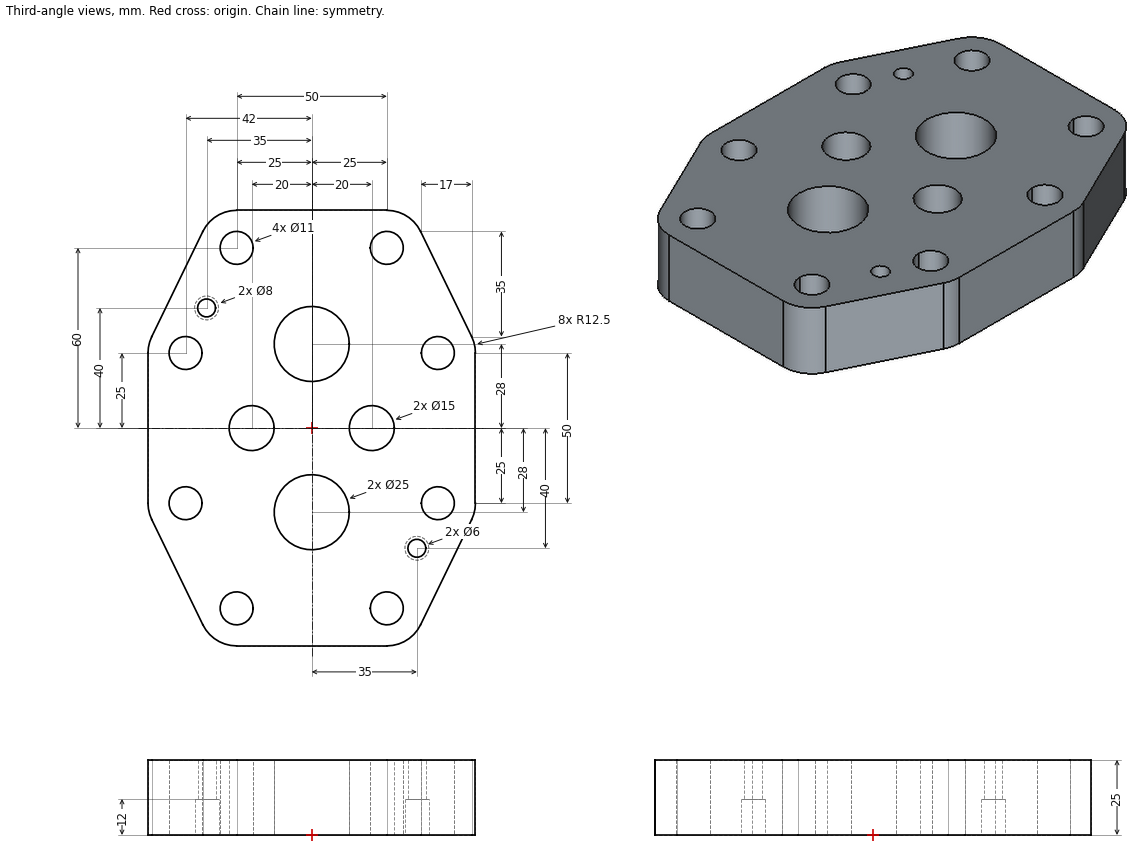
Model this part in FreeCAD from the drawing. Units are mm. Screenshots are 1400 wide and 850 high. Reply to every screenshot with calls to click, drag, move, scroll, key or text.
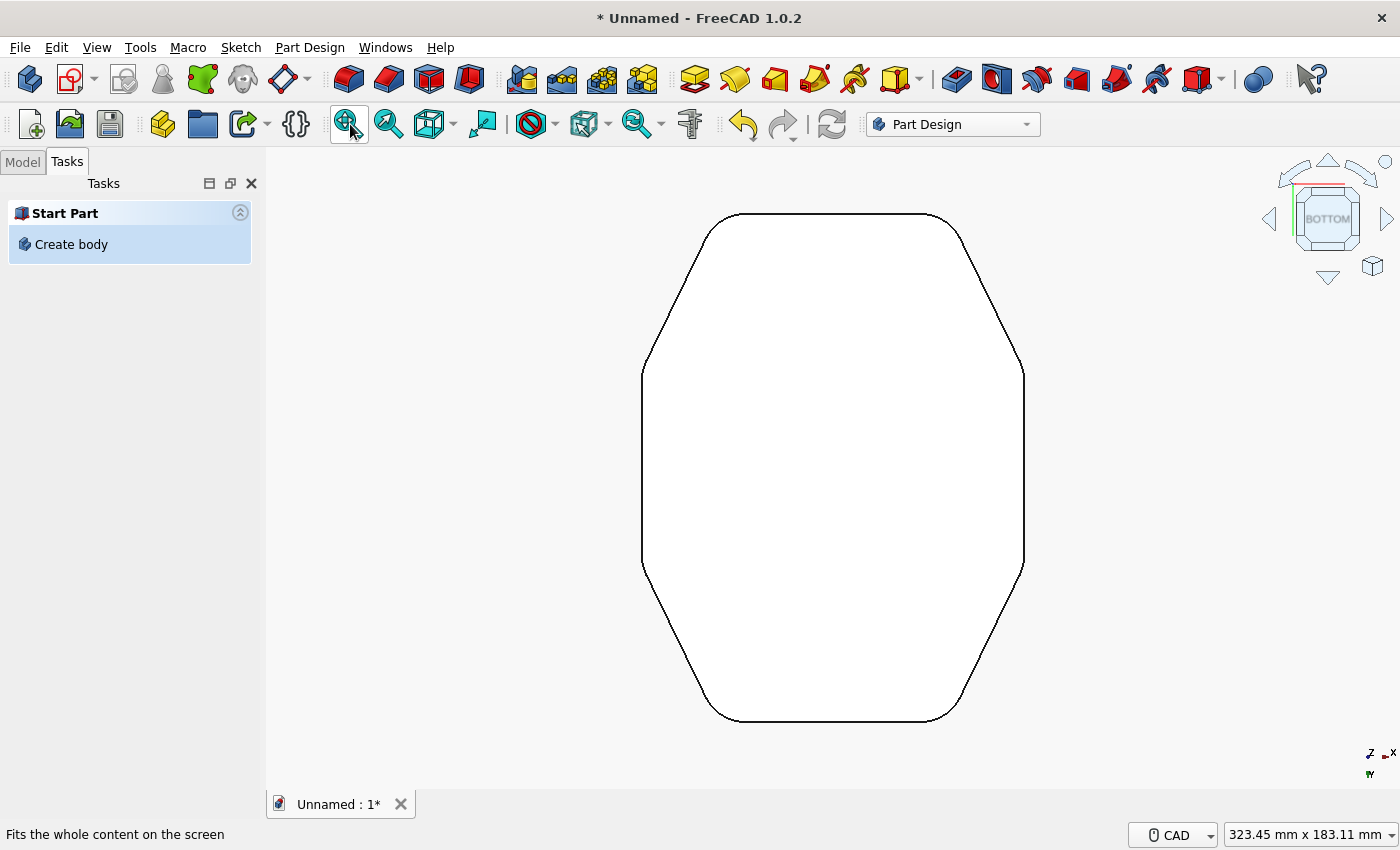
click(833, 467)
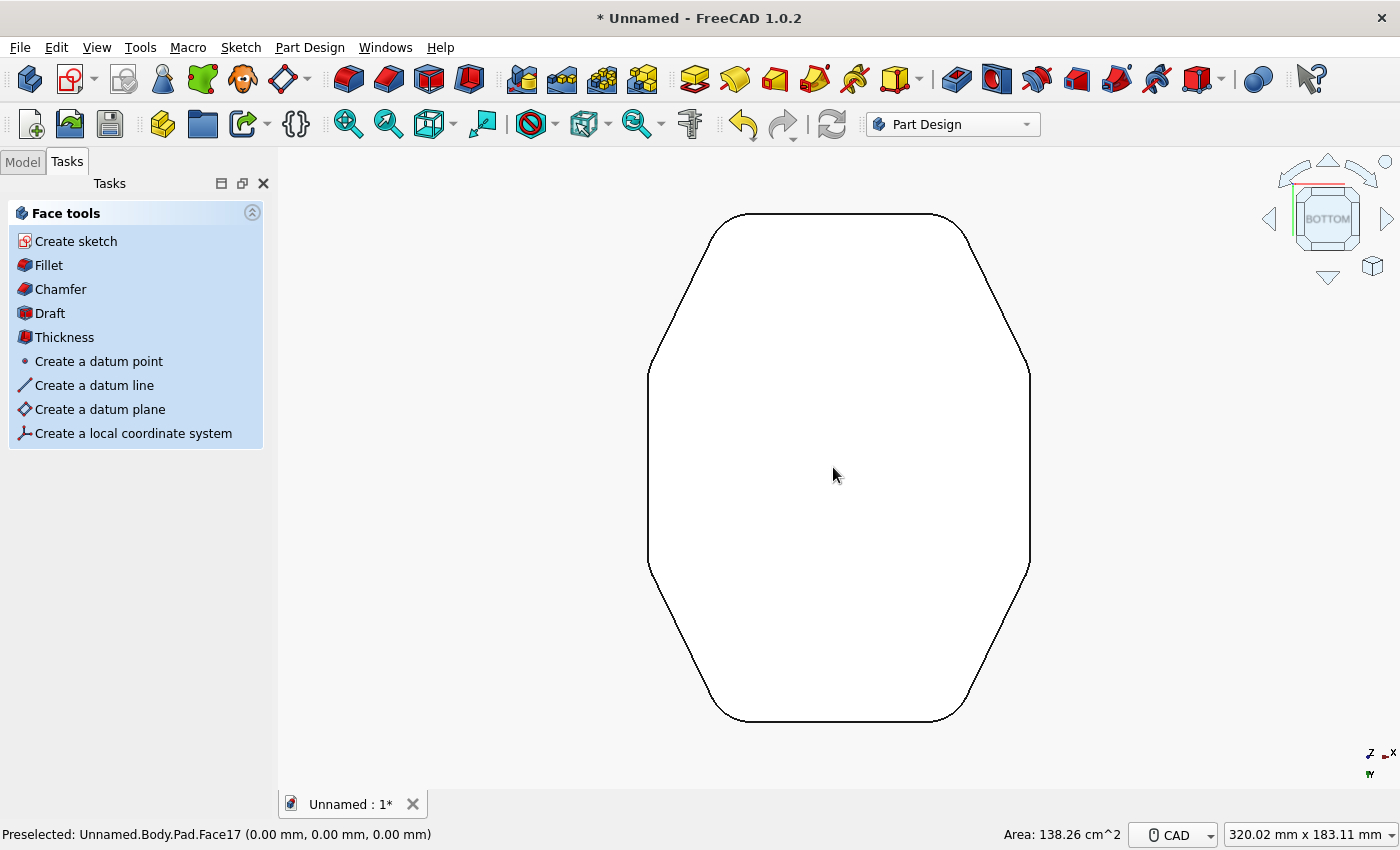
click(70, 80)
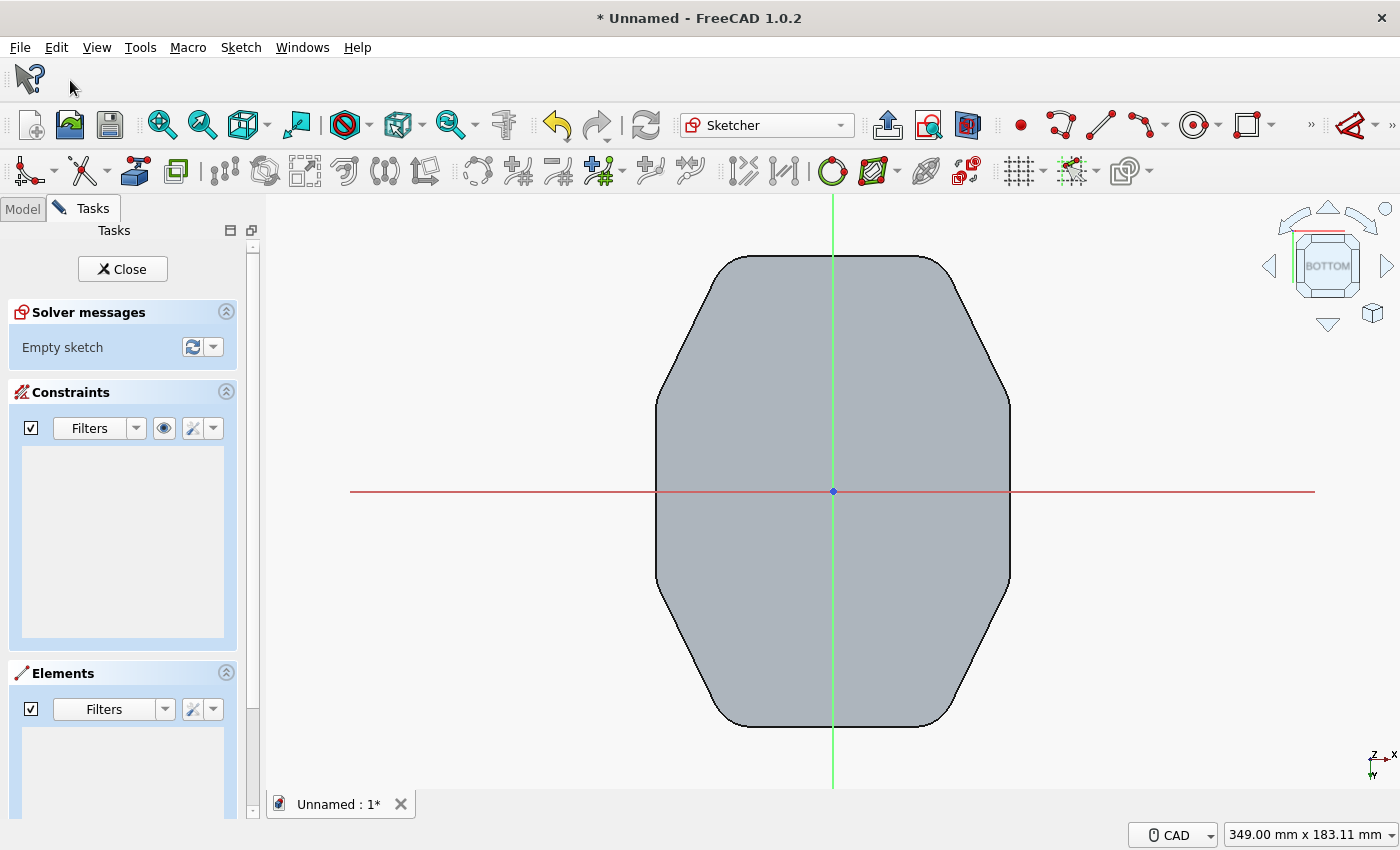
click(1194, 126)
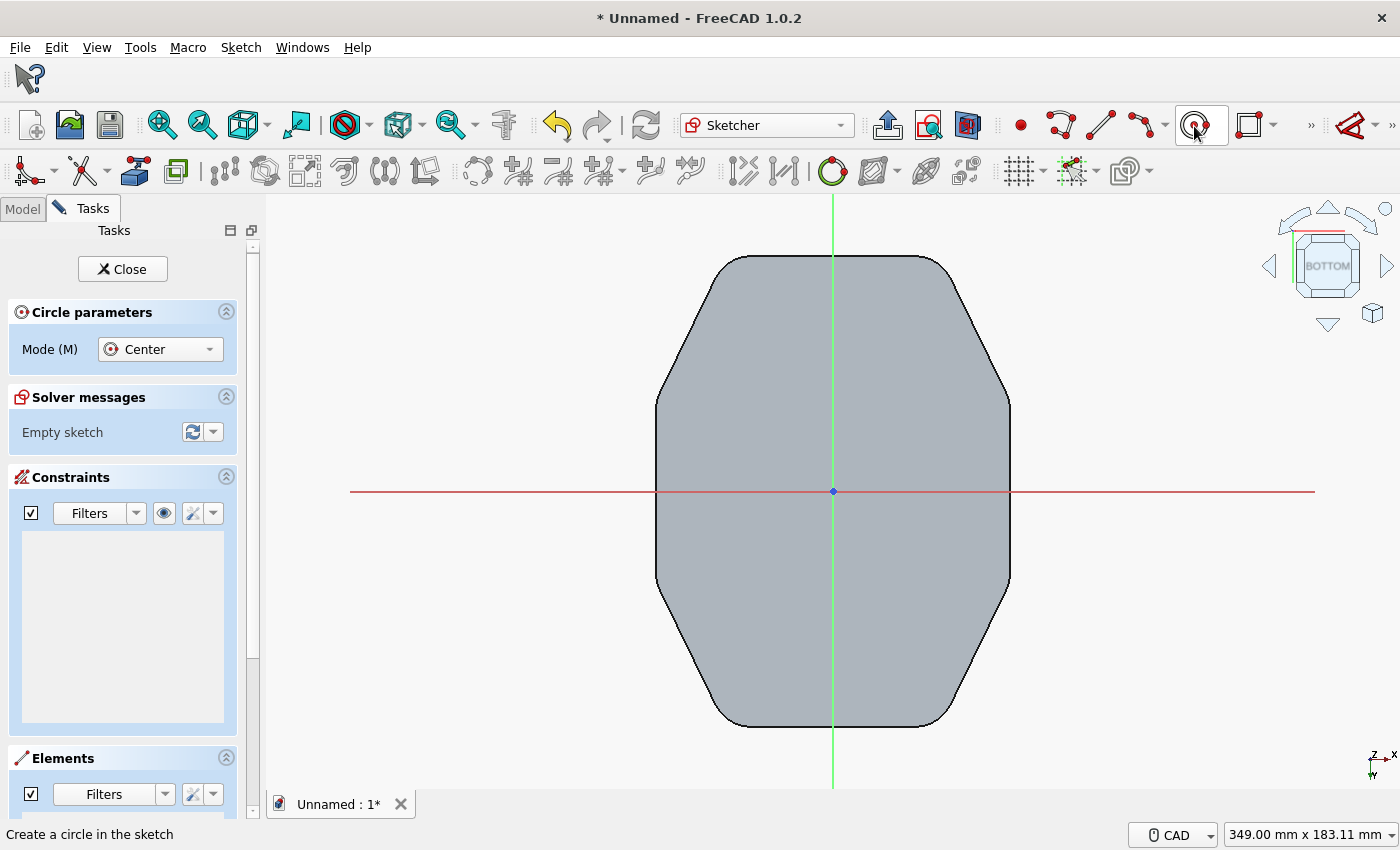
scroll(752, 686, up, 2)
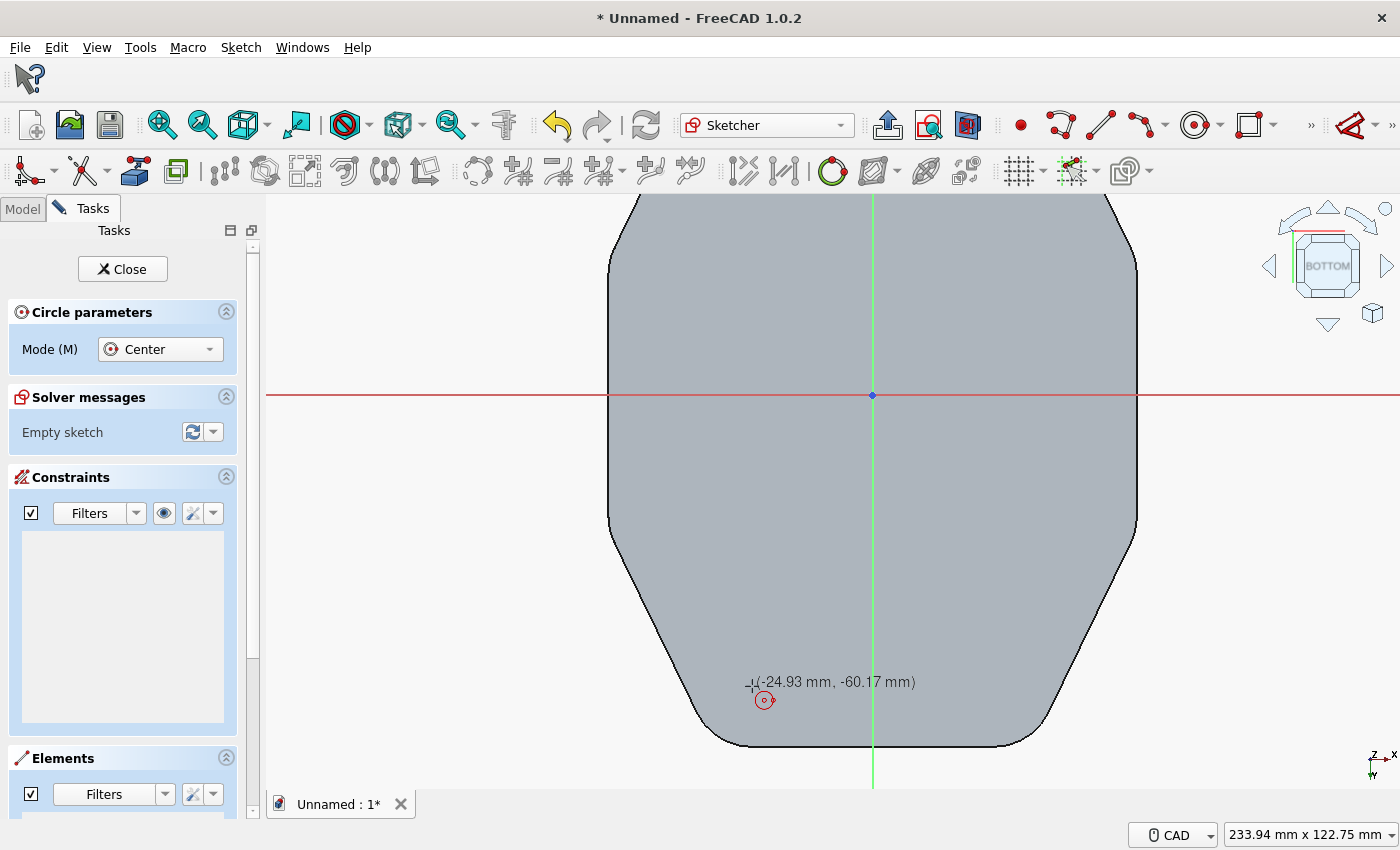
click(751, 686)
click(770, 667)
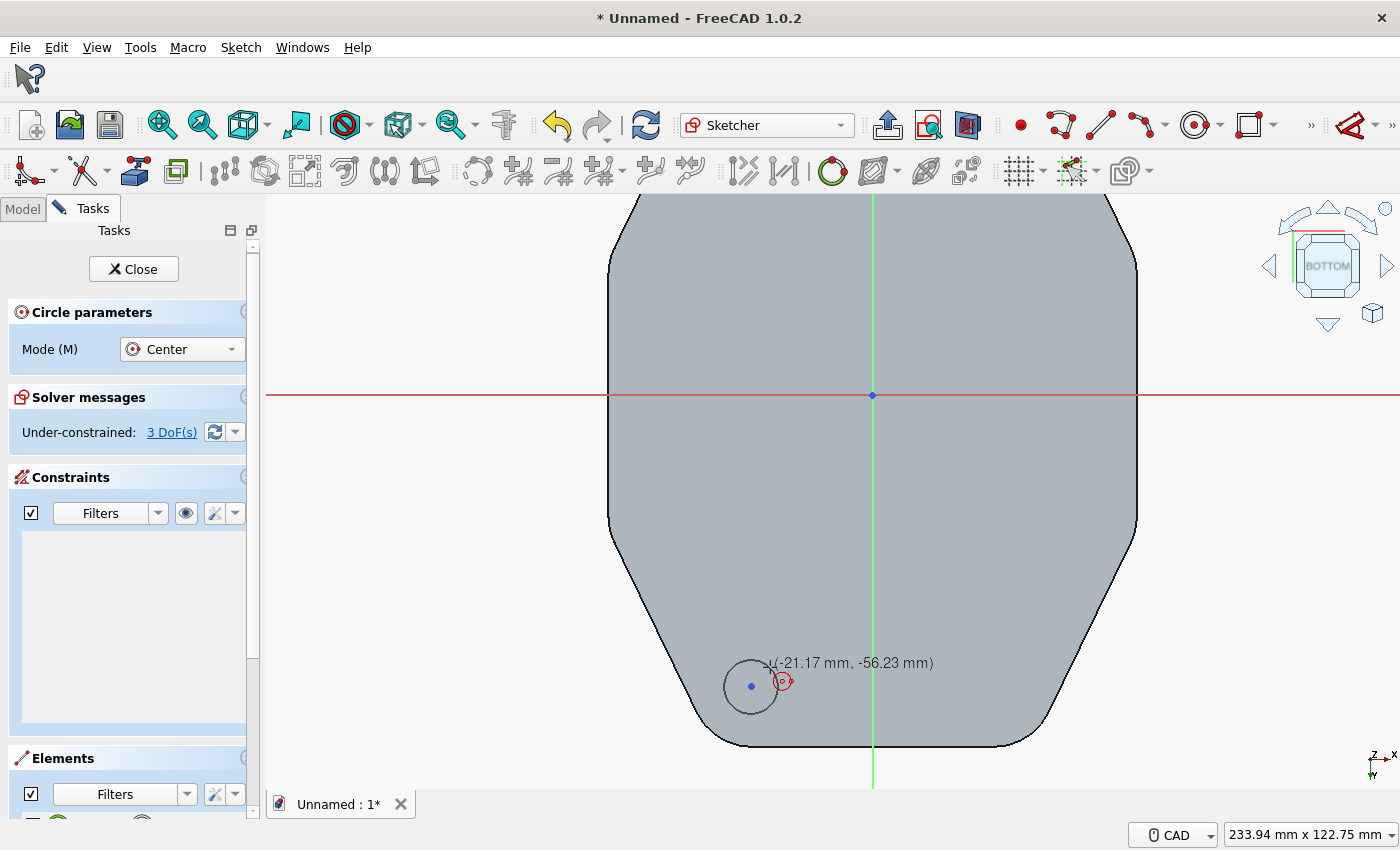
click(669, 517)
click(688, 498)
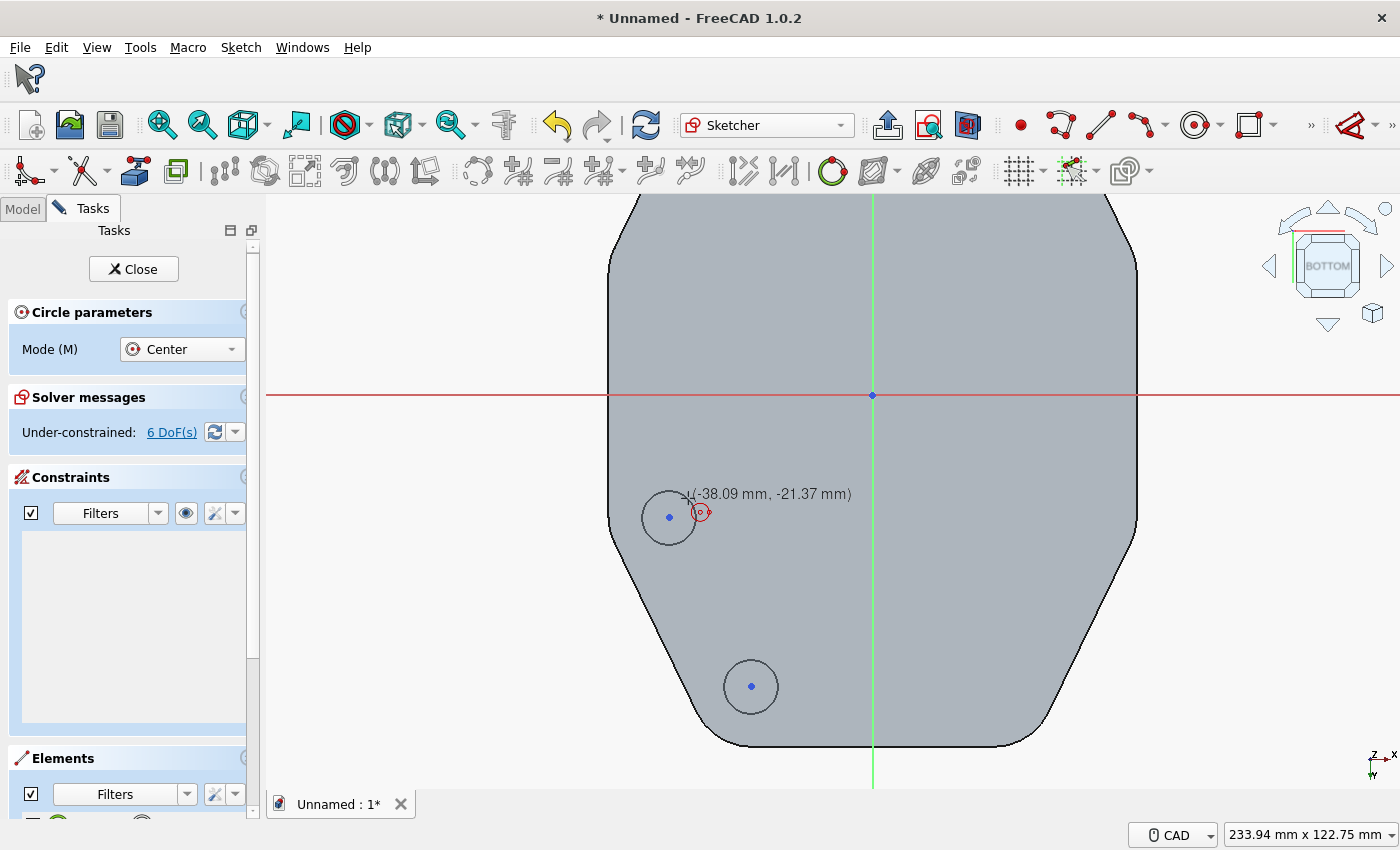
click(669, 274)
click(688, 255)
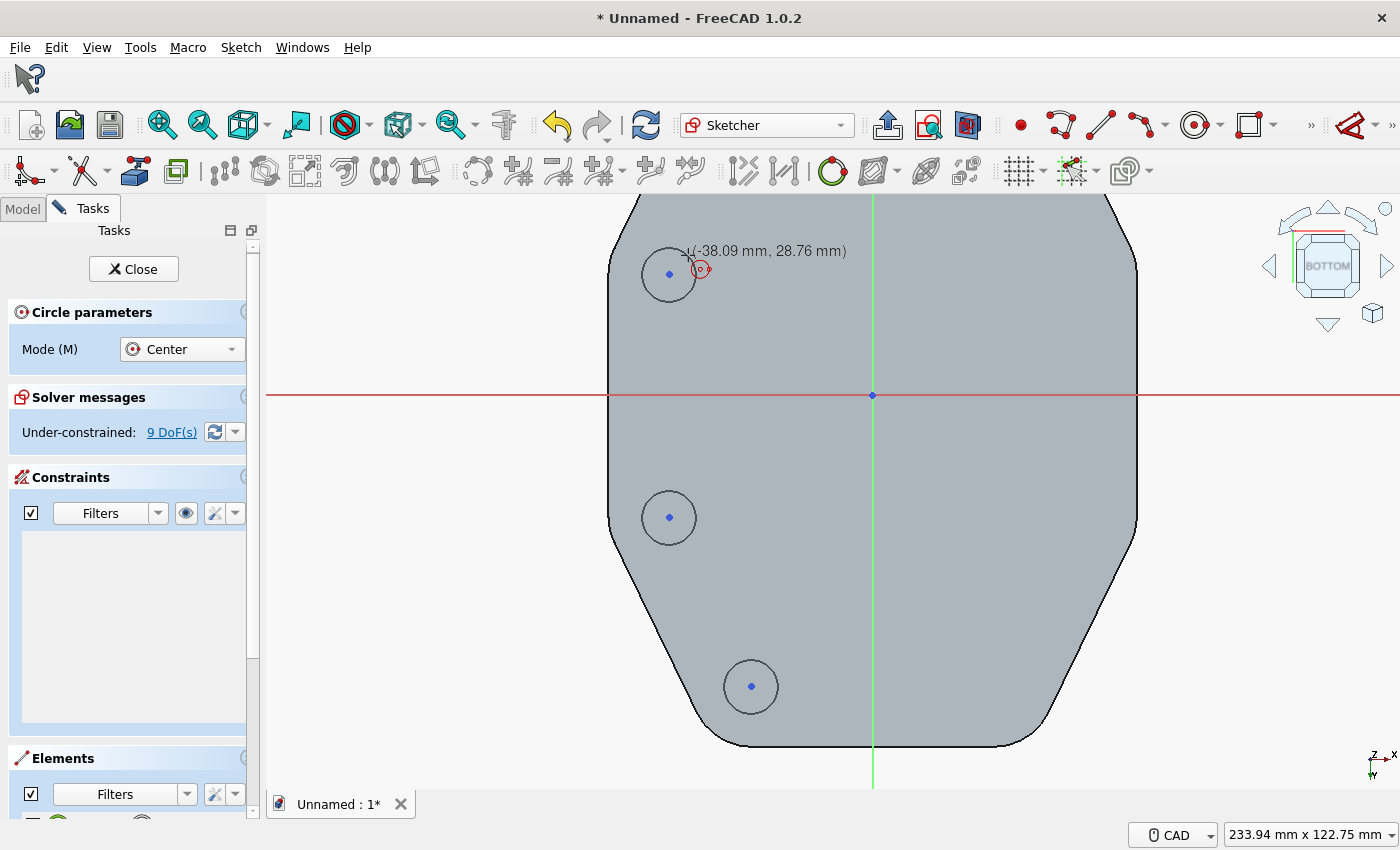
click(873, 260)